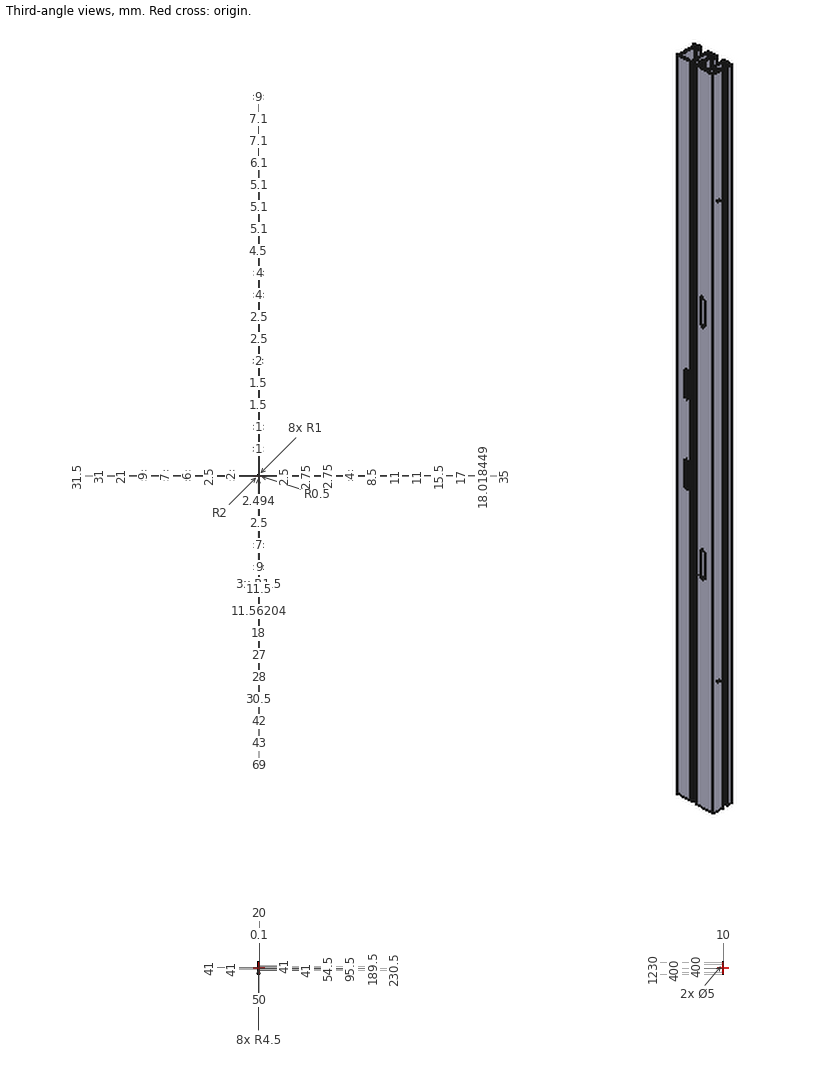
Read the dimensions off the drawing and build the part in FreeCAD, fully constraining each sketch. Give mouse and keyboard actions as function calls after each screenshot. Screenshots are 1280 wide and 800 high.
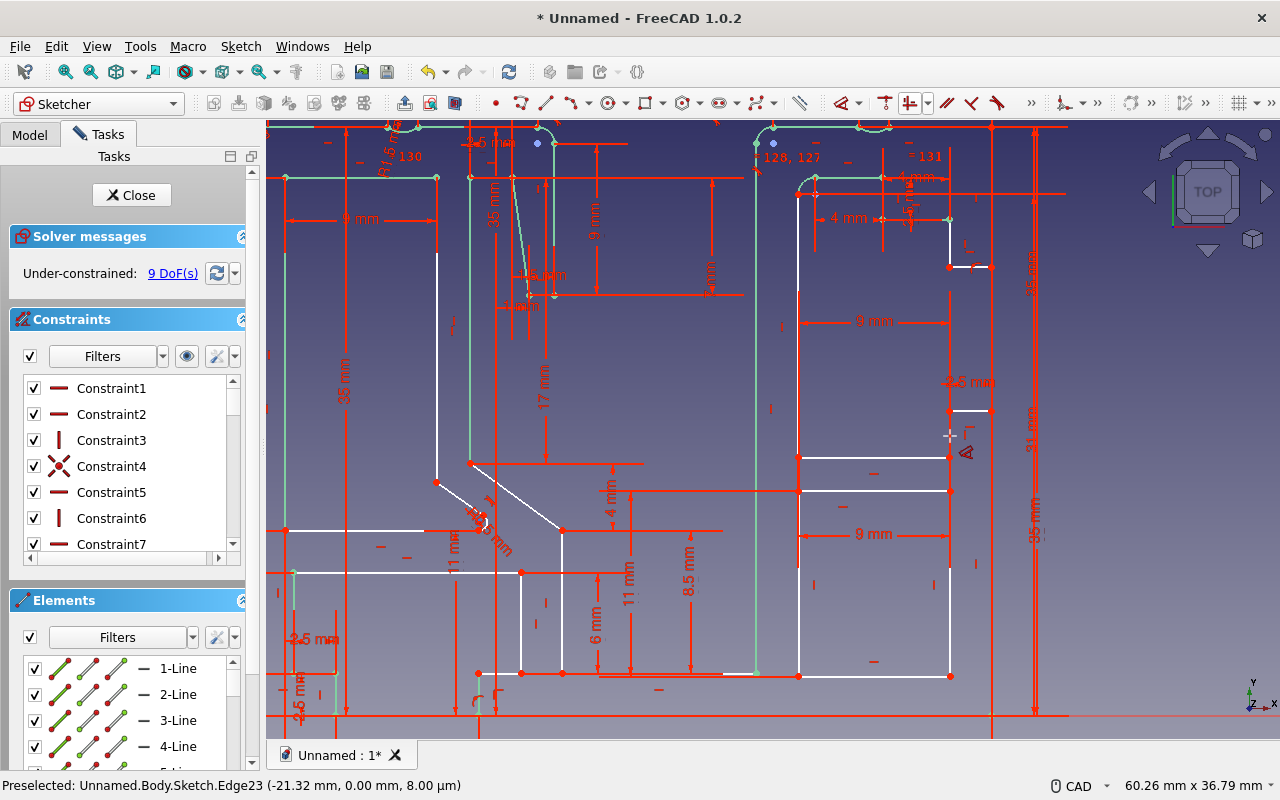
click(950, 434)
click(916, 434)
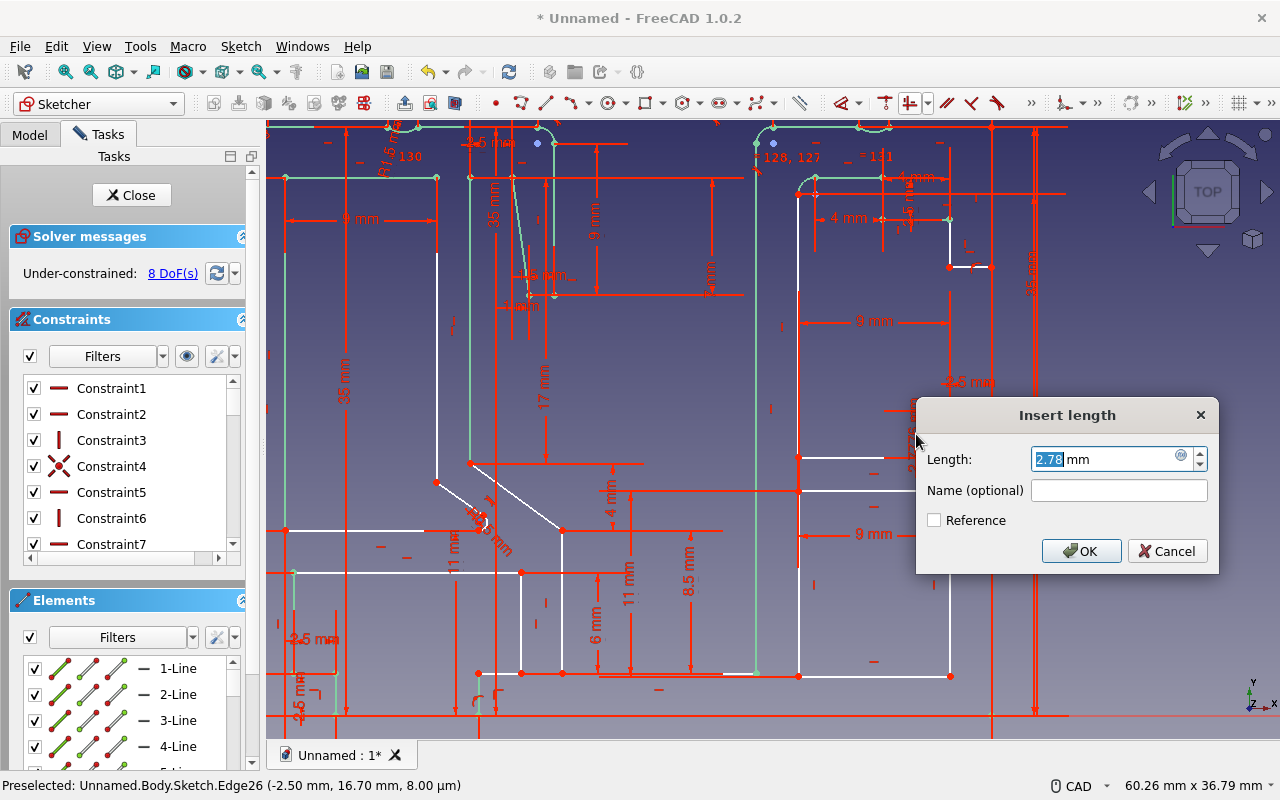
text(2.75)
key(Return)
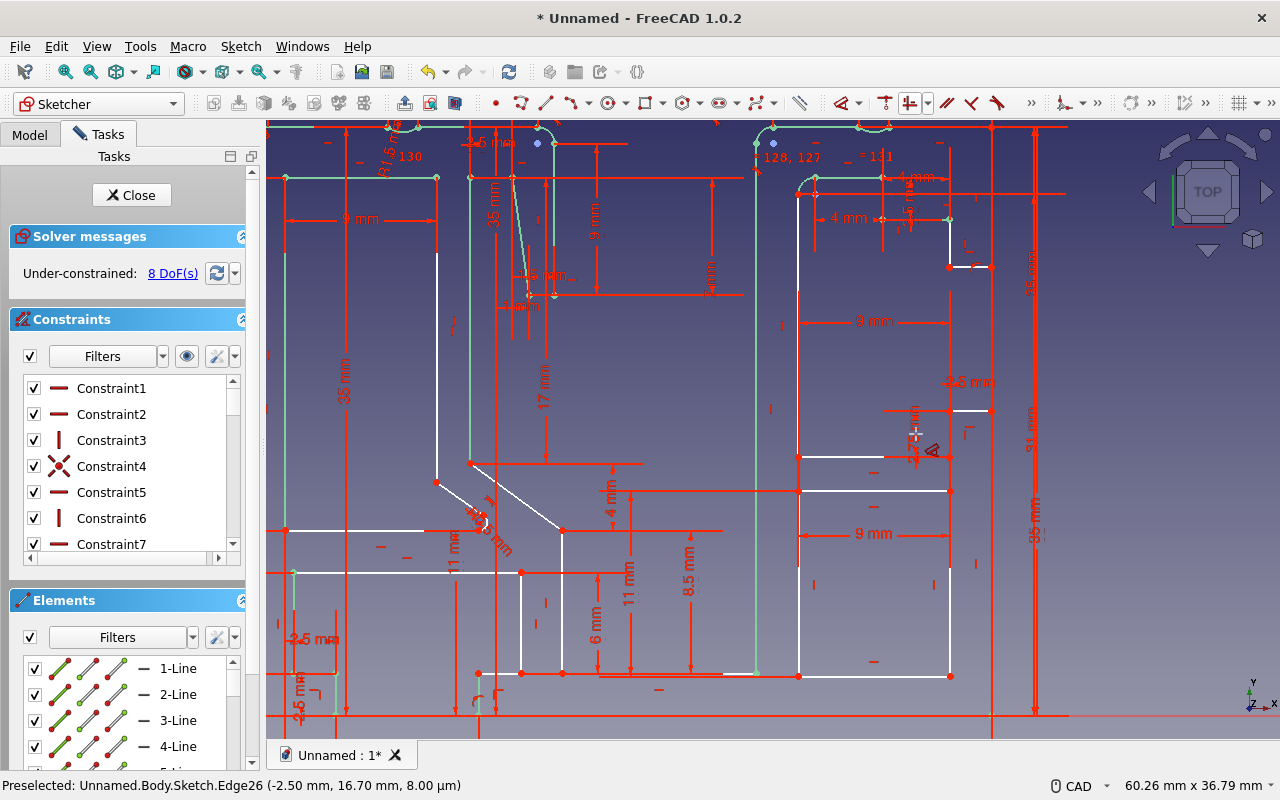
click(798, 378)
click(832, 326)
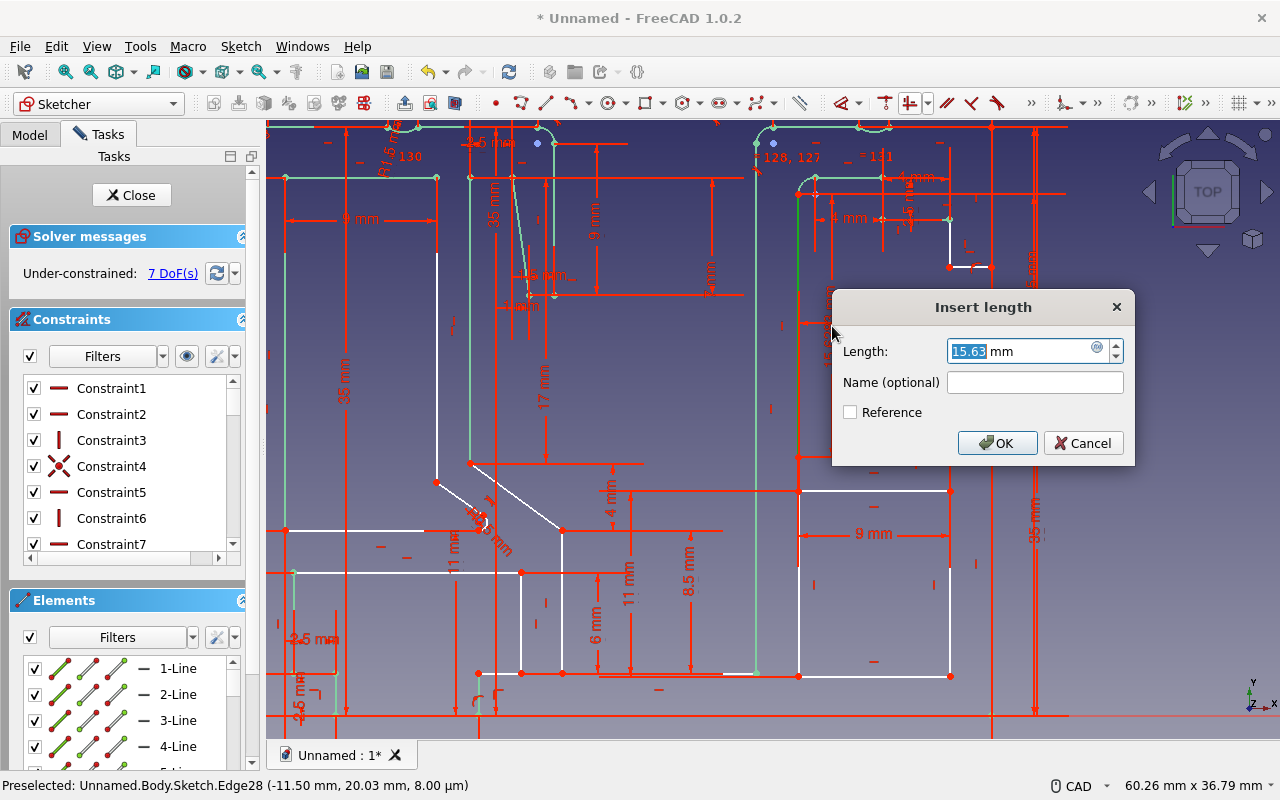
text(15.5)
key(Return)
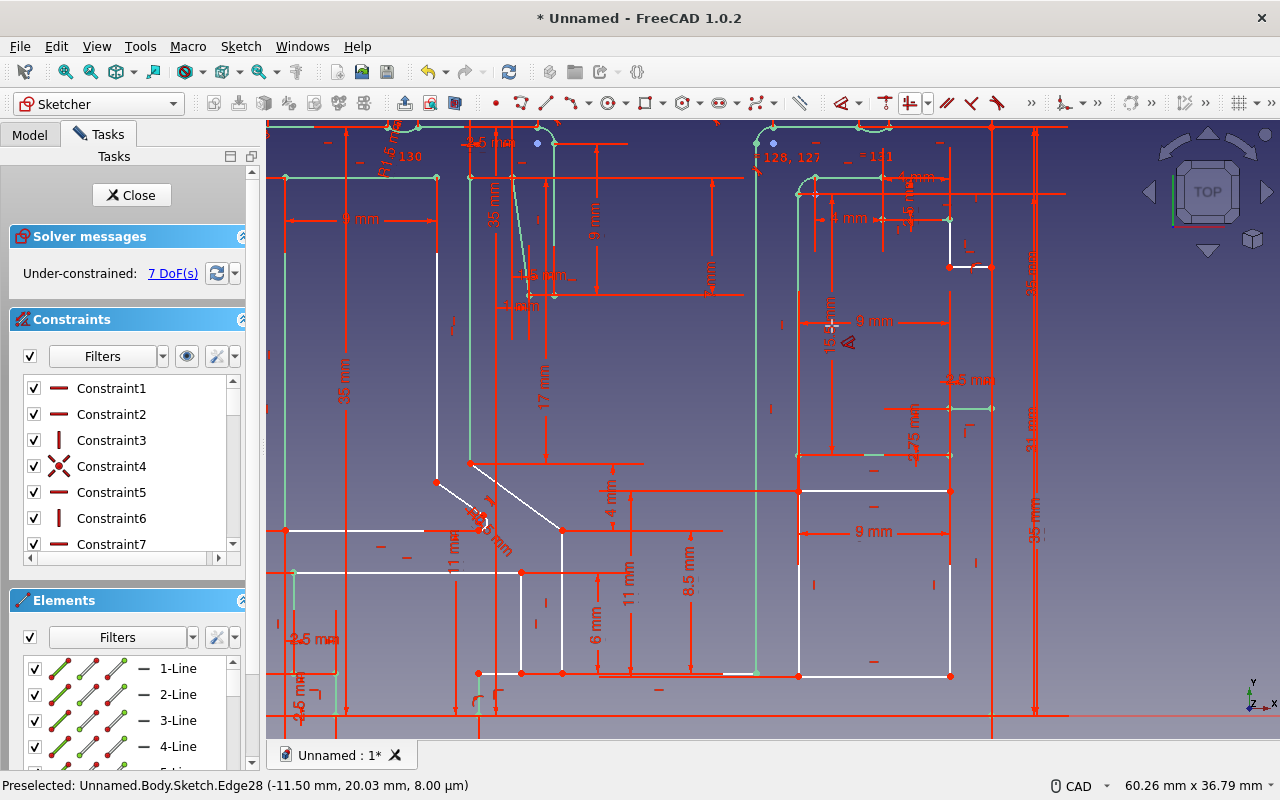
click(950, 234)
click(916, 243)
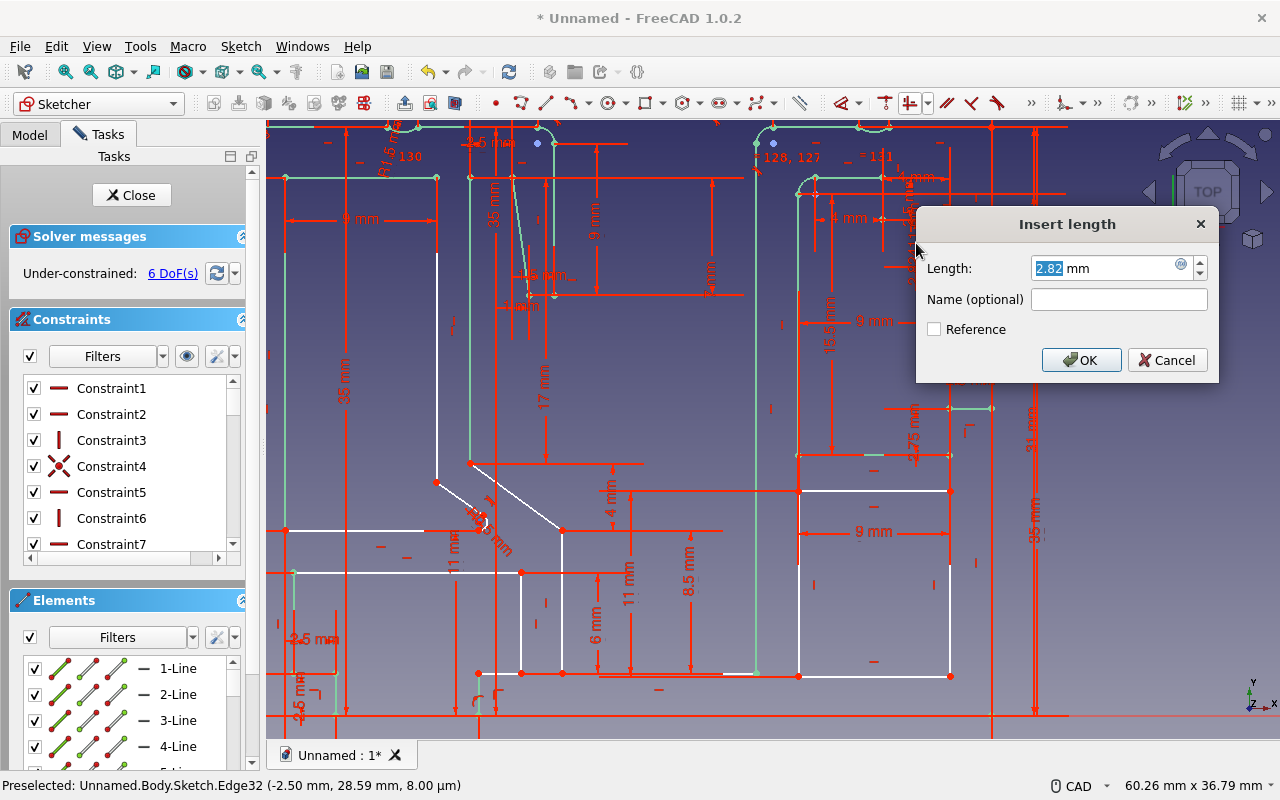
text(2.75)
key(Return)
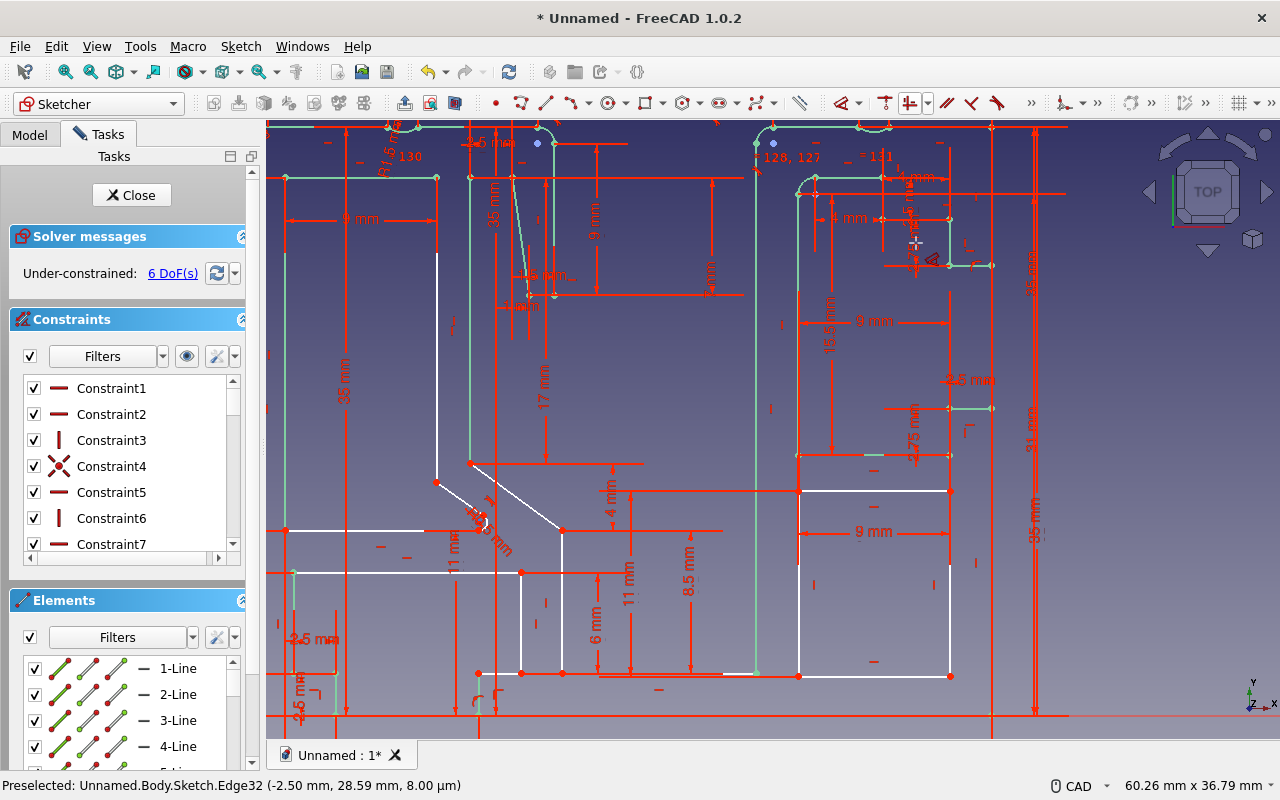
click(698, 674)
click(704, 640)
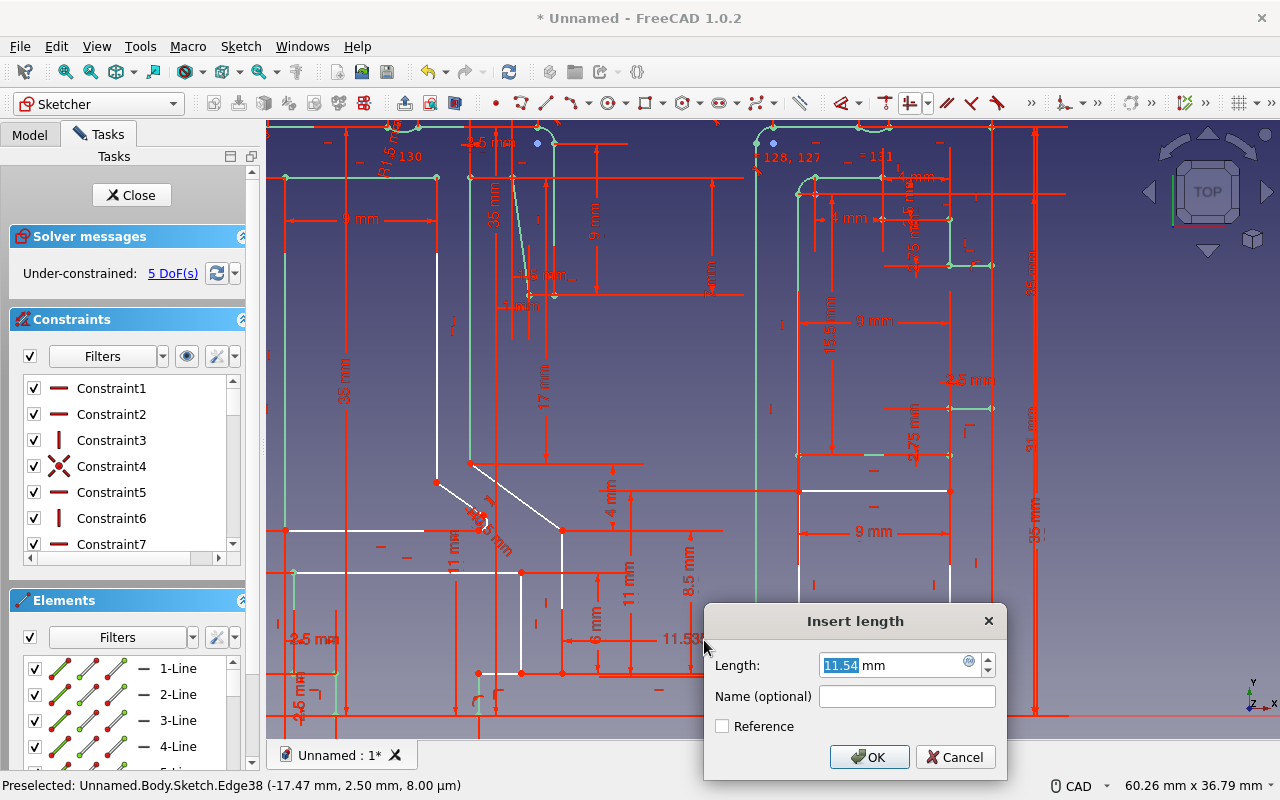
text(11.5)
key(Return)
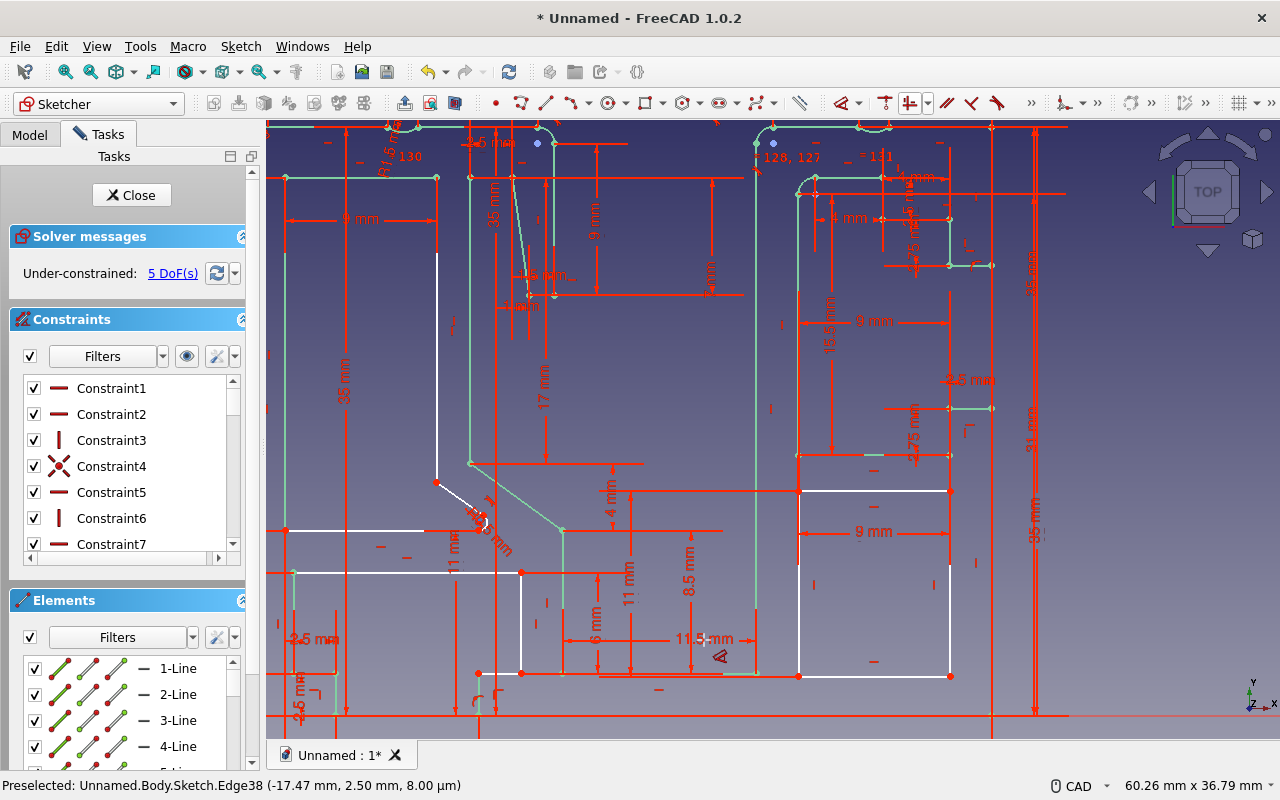
click(799, 677)
click(1026, 694)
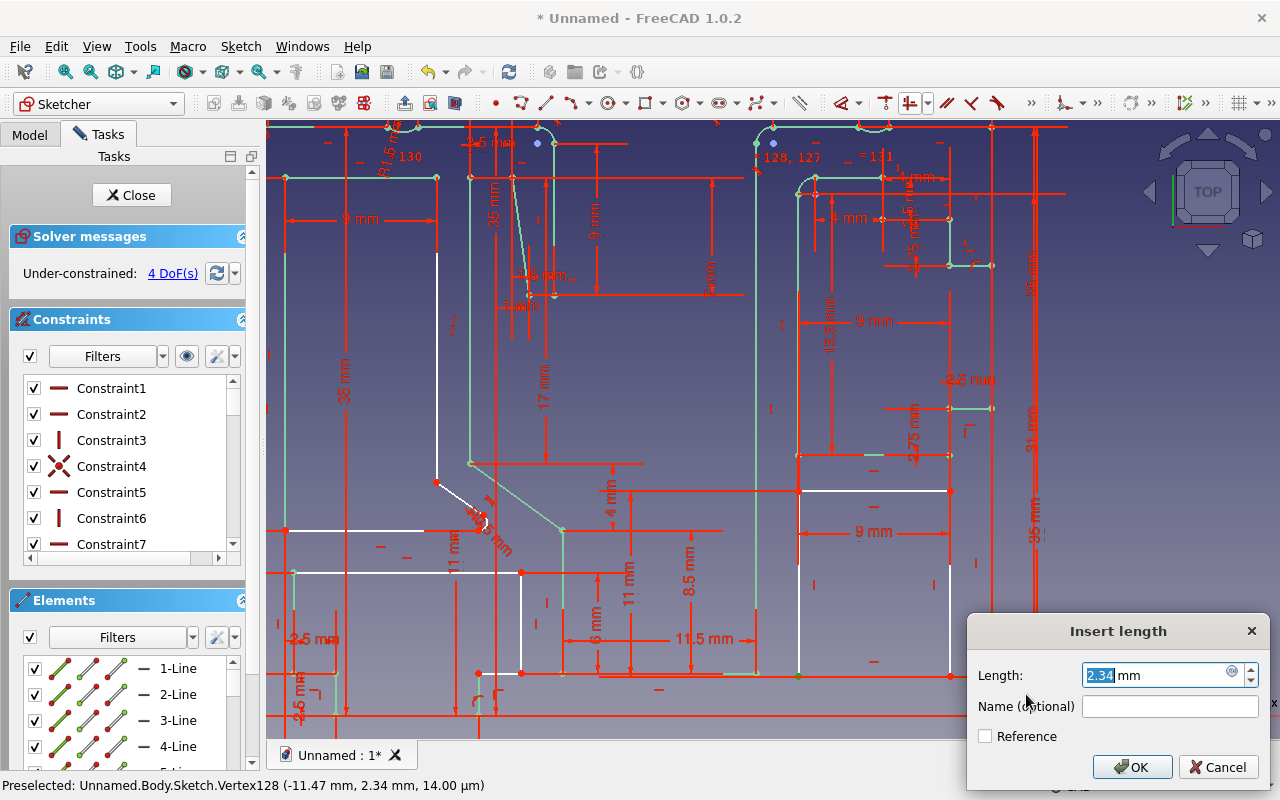
text(2.5)
key(Return)